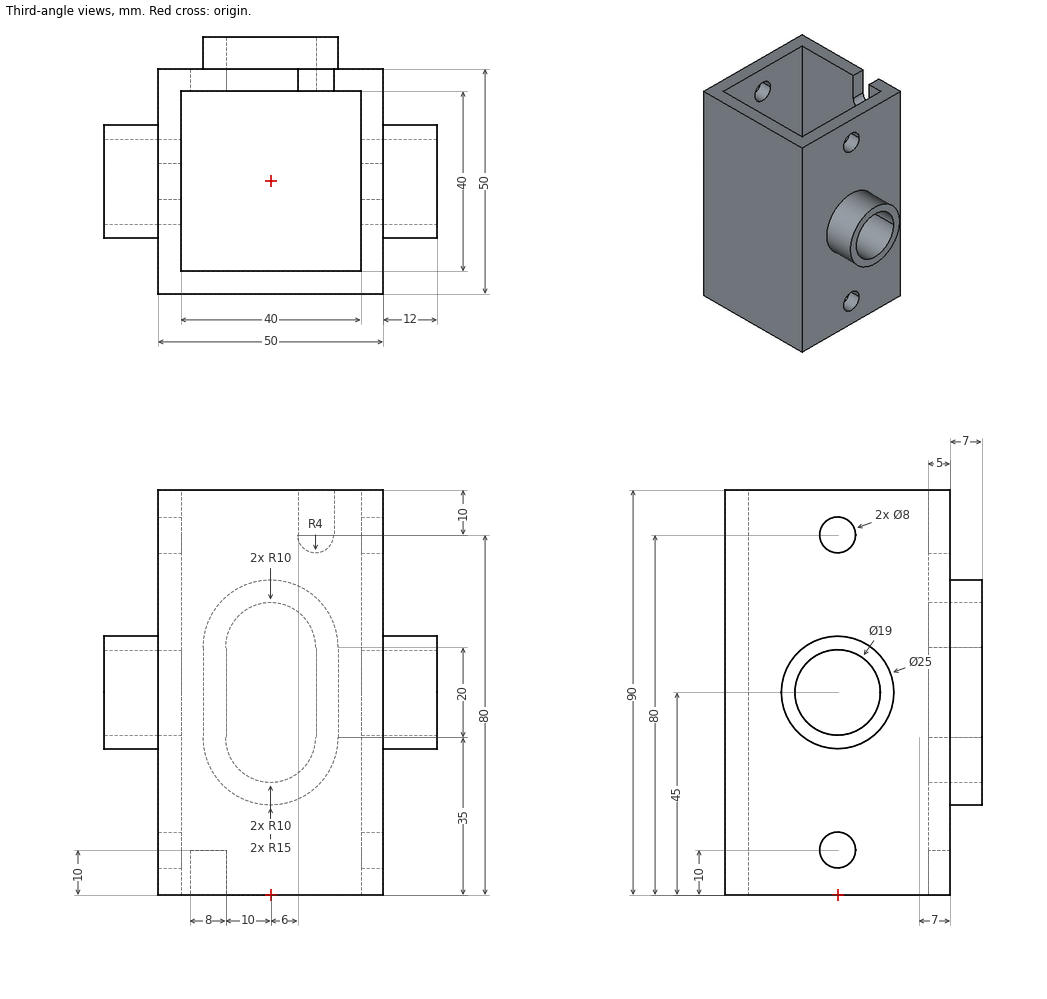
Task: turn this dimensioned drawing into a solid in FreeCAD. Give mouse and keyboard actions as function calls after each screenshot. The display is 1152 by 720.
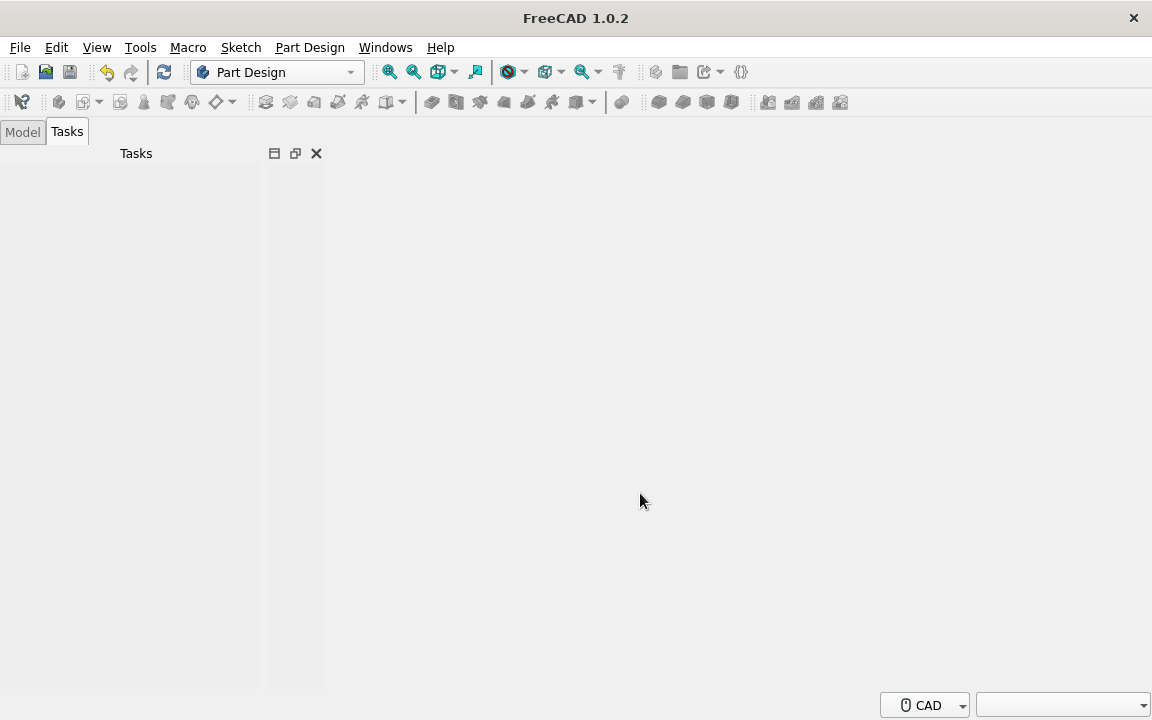
key(ctrl+n)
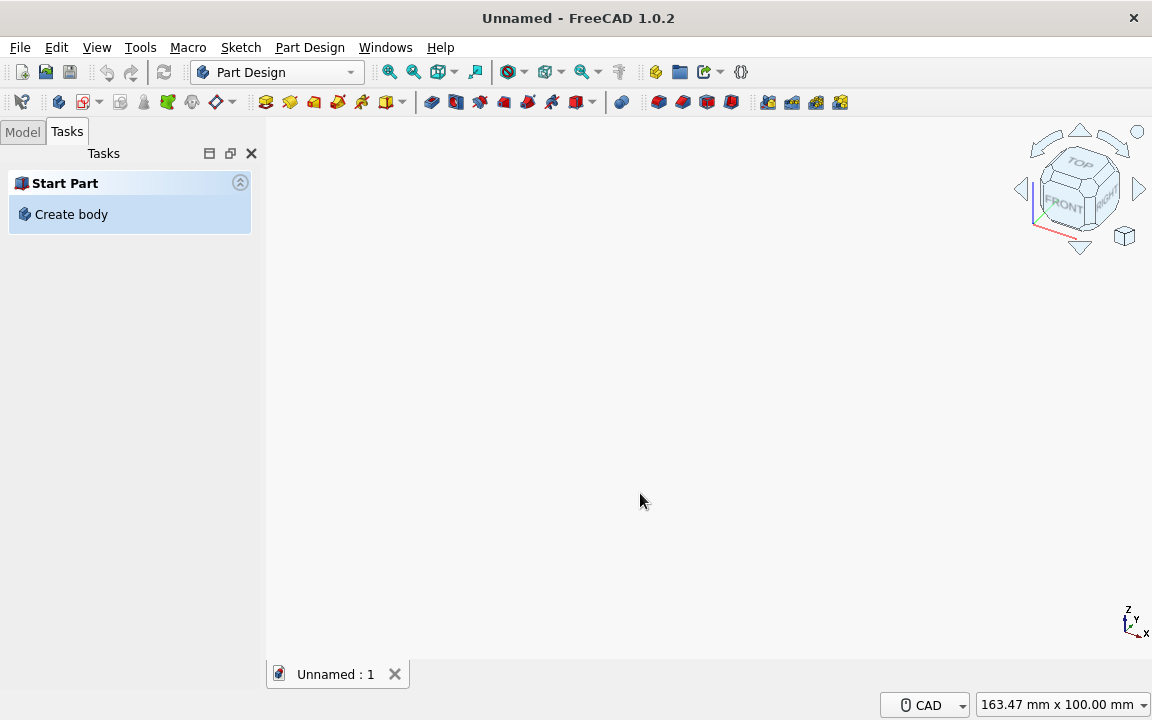
click(84, 102)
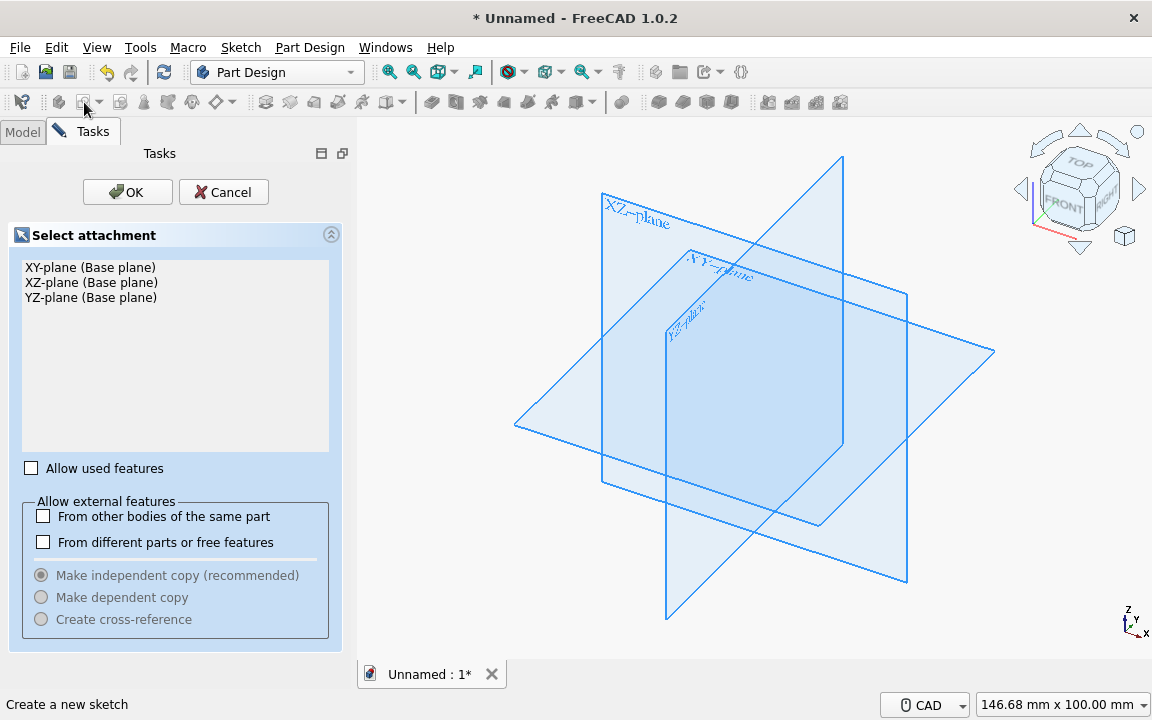
click(82, 268)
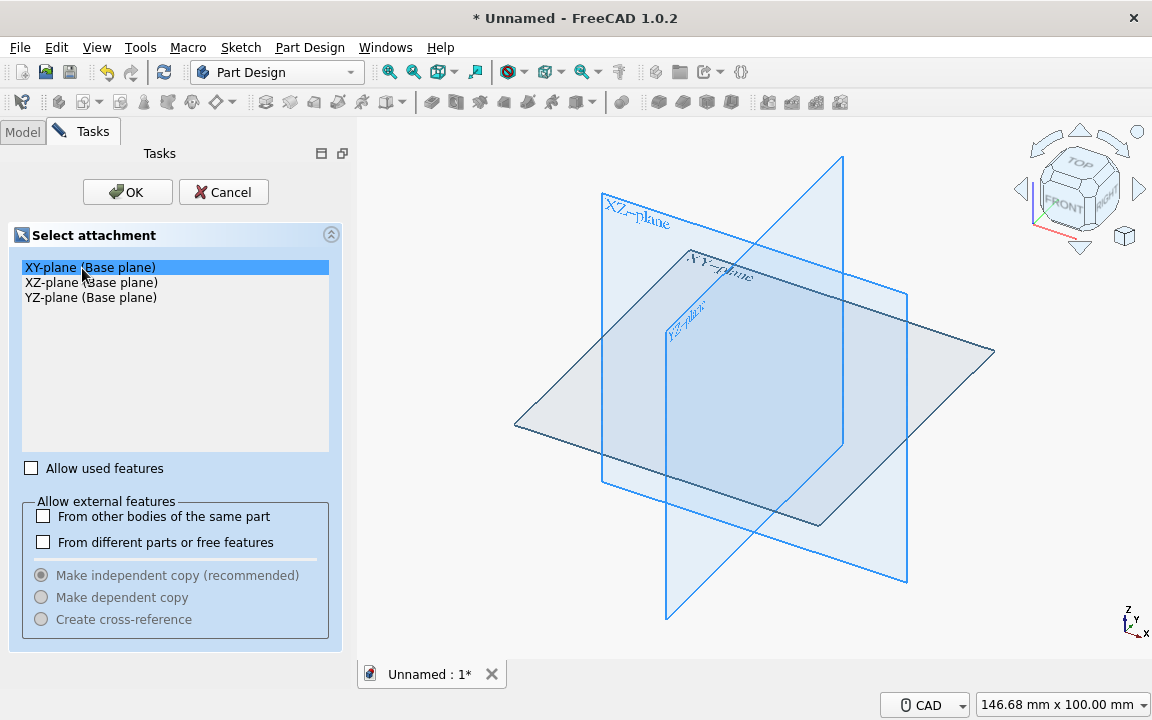
click(128, 192)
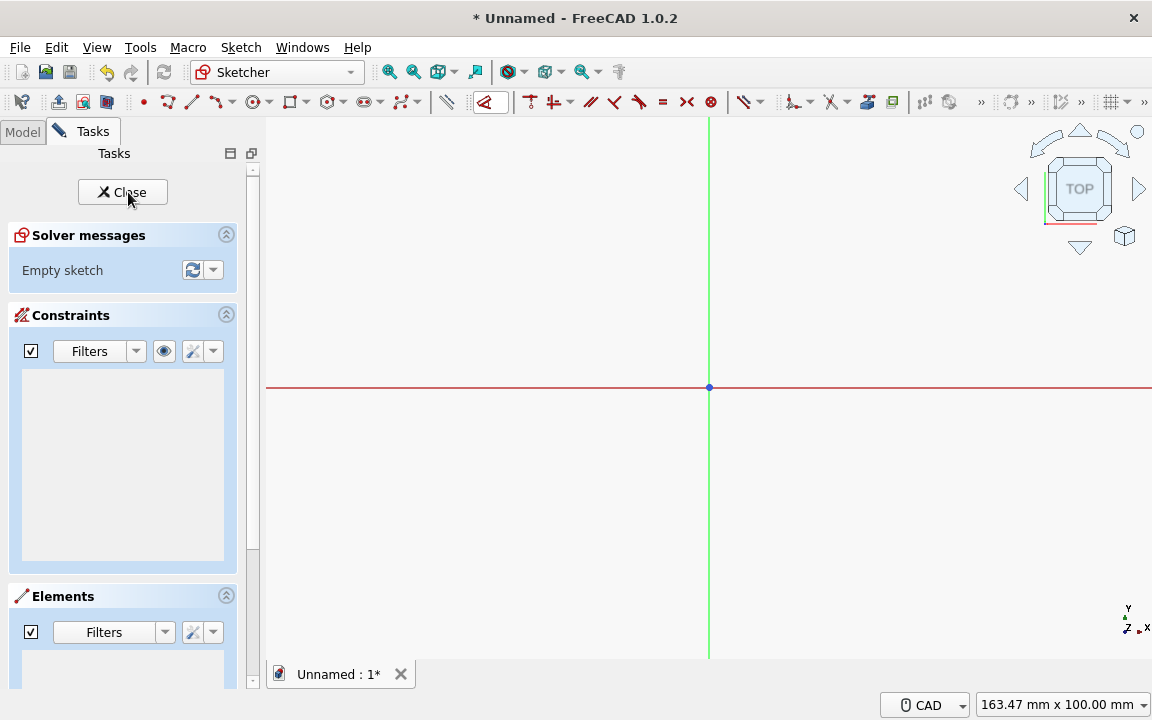
key(g)
key(v)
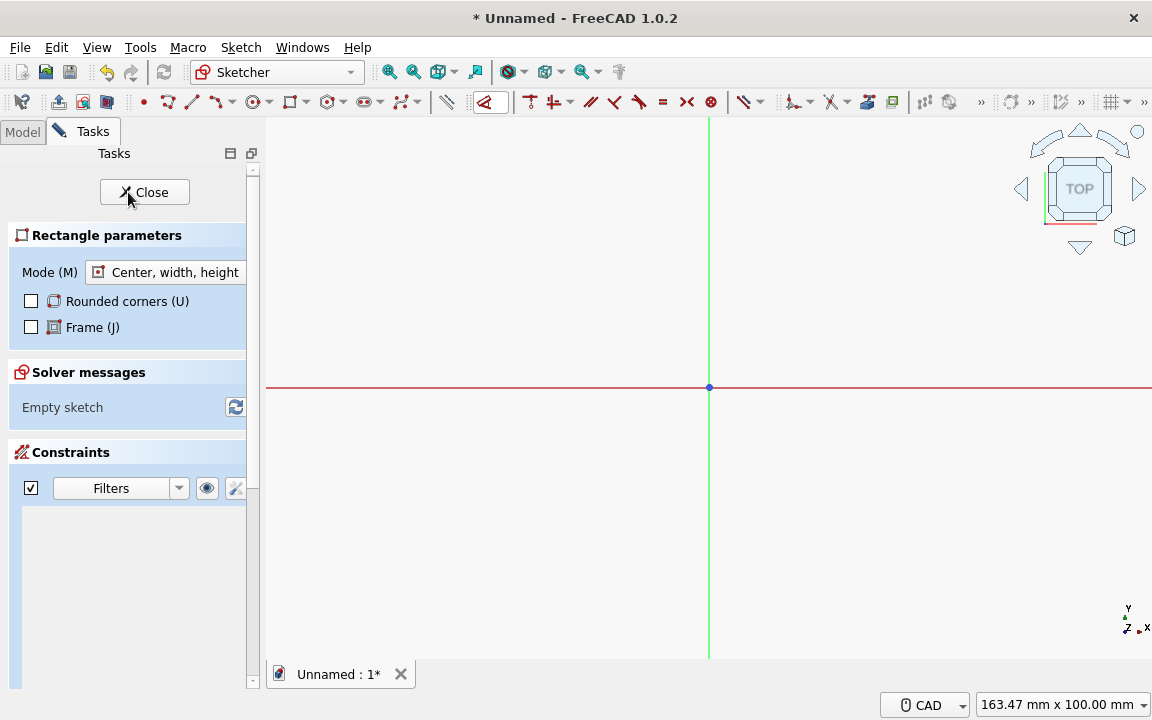
click(709, 388)
click(844, 252)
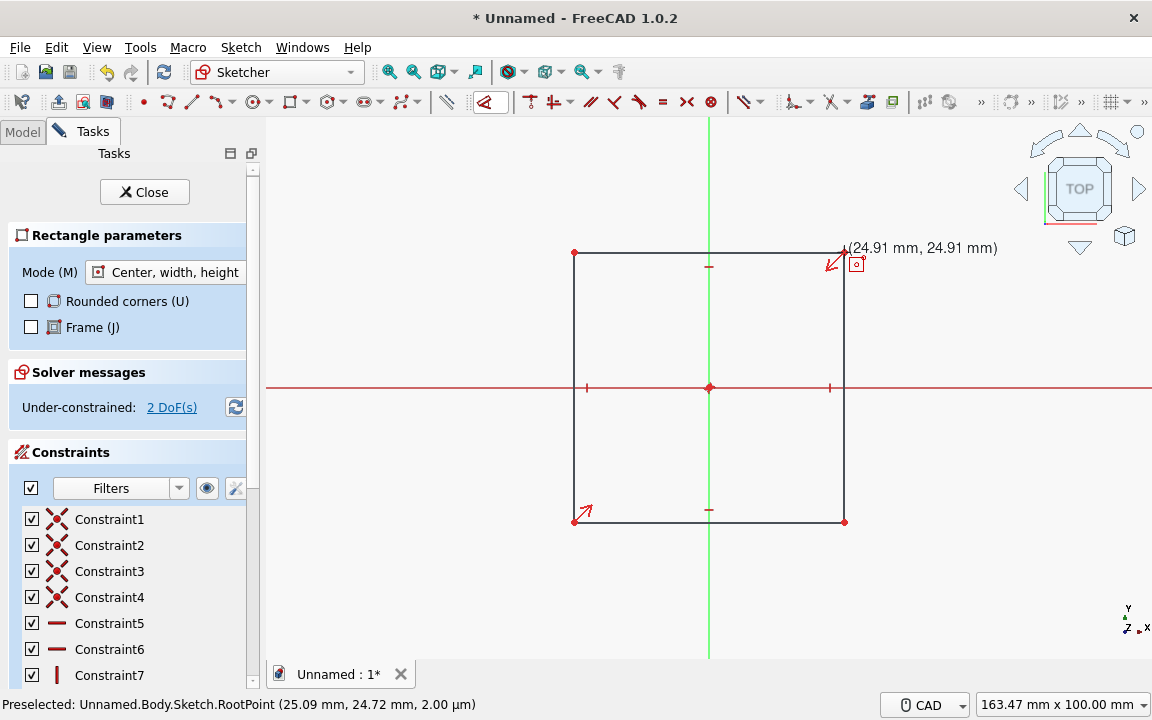
click(709, 388)
click(817, 280)
key(Escape)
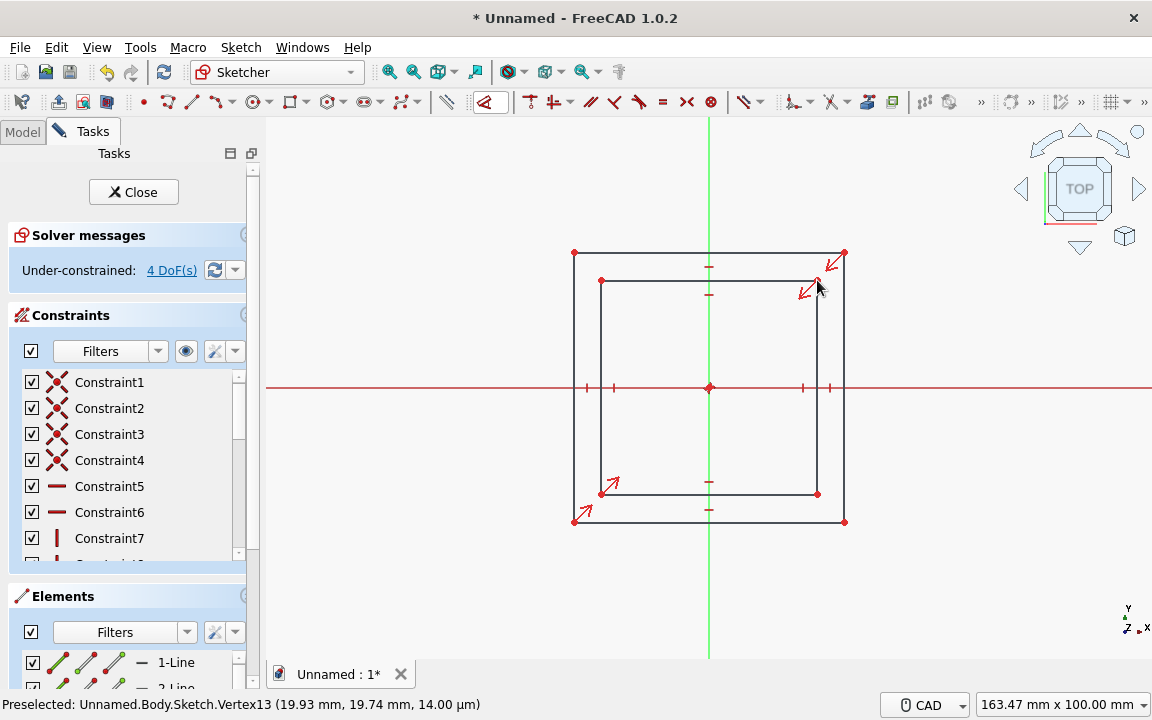
key(d)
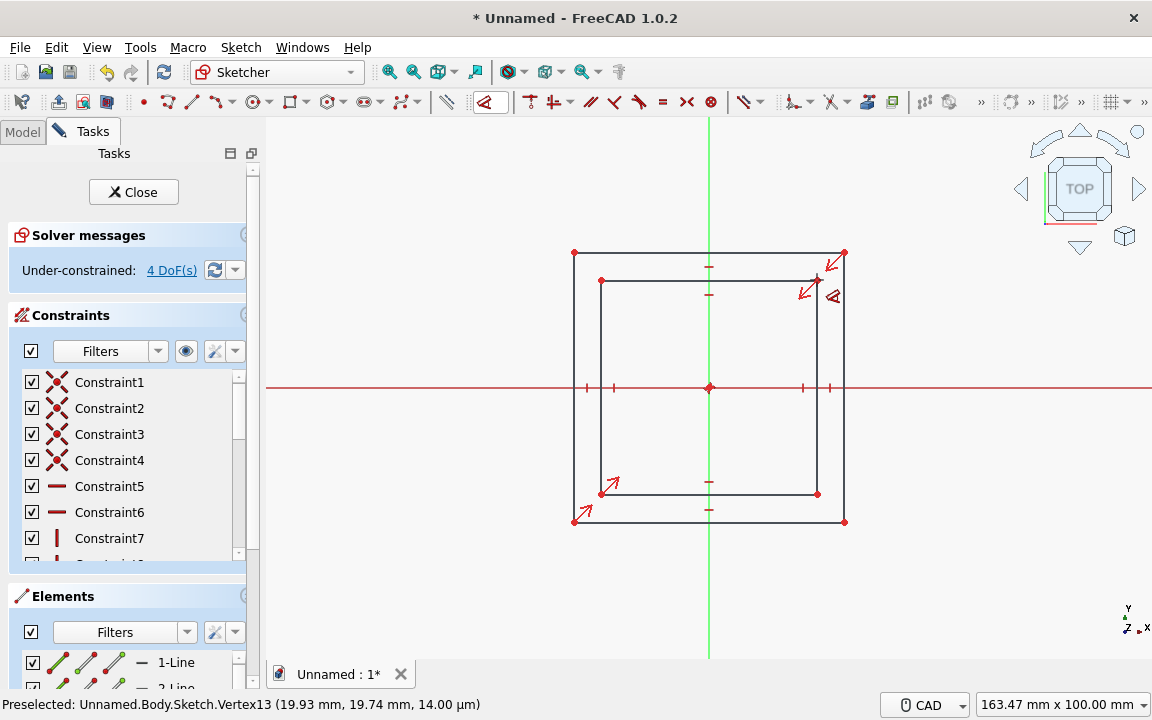
click(655, 523)
click(647, 557)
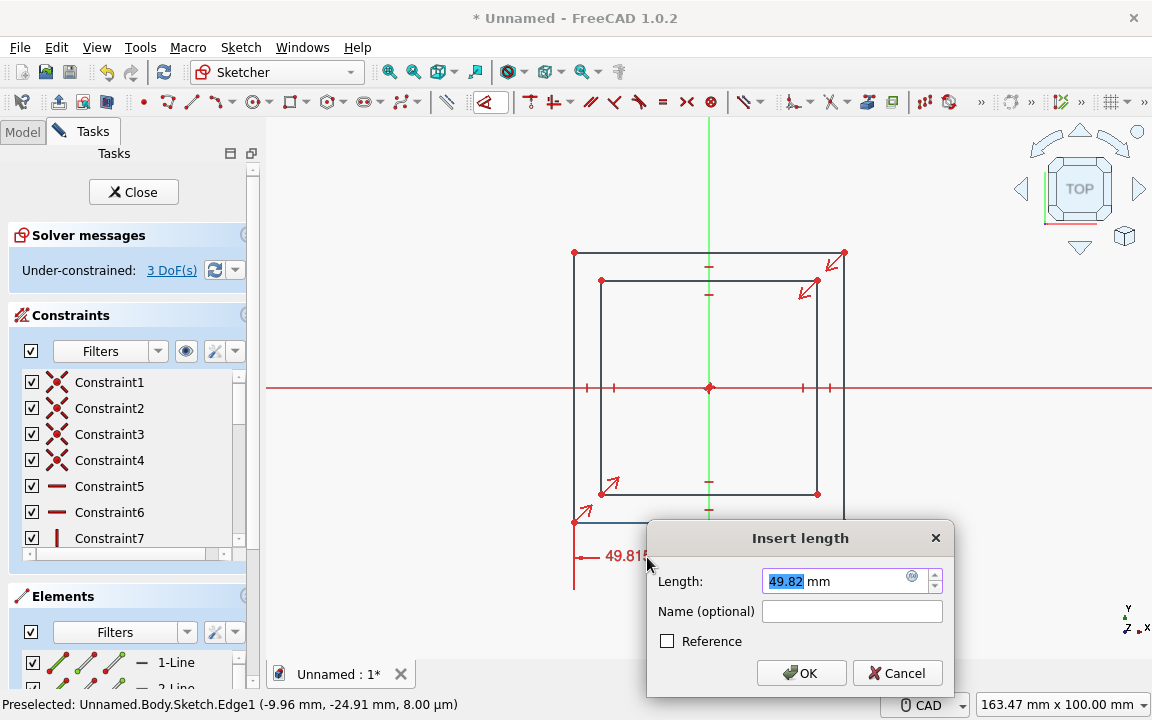
text(50)
key(Return)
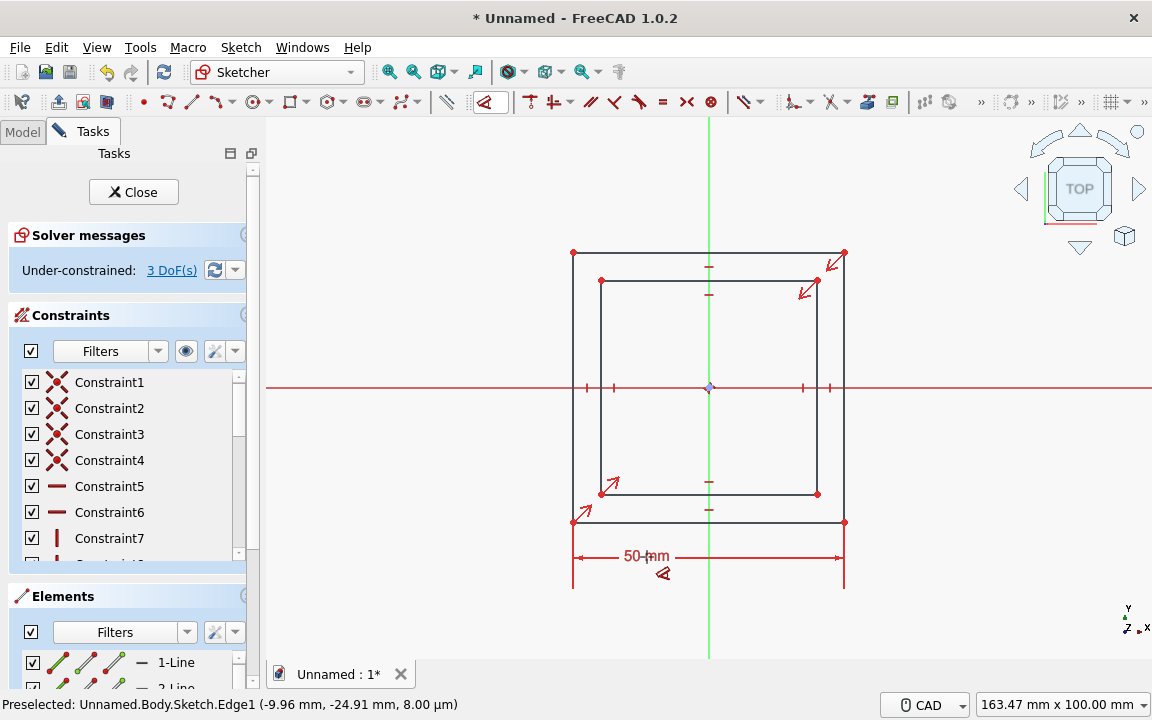
click(844, 442)
click(878, 326)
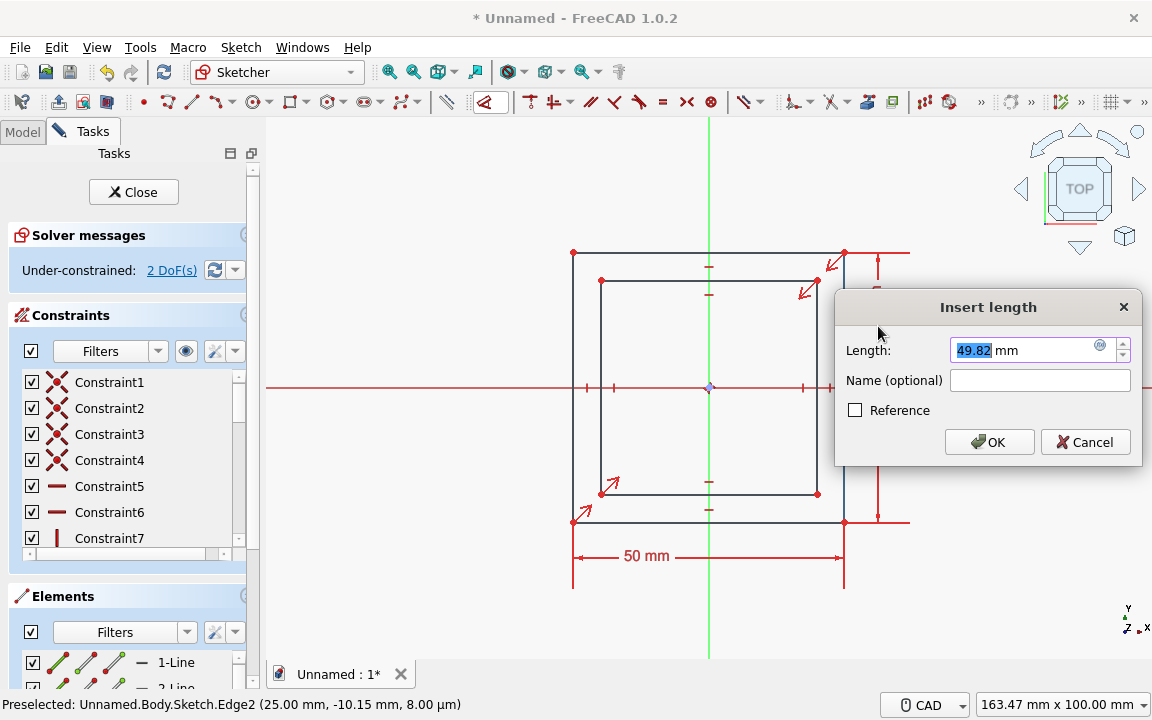
text(50)
key(Return)